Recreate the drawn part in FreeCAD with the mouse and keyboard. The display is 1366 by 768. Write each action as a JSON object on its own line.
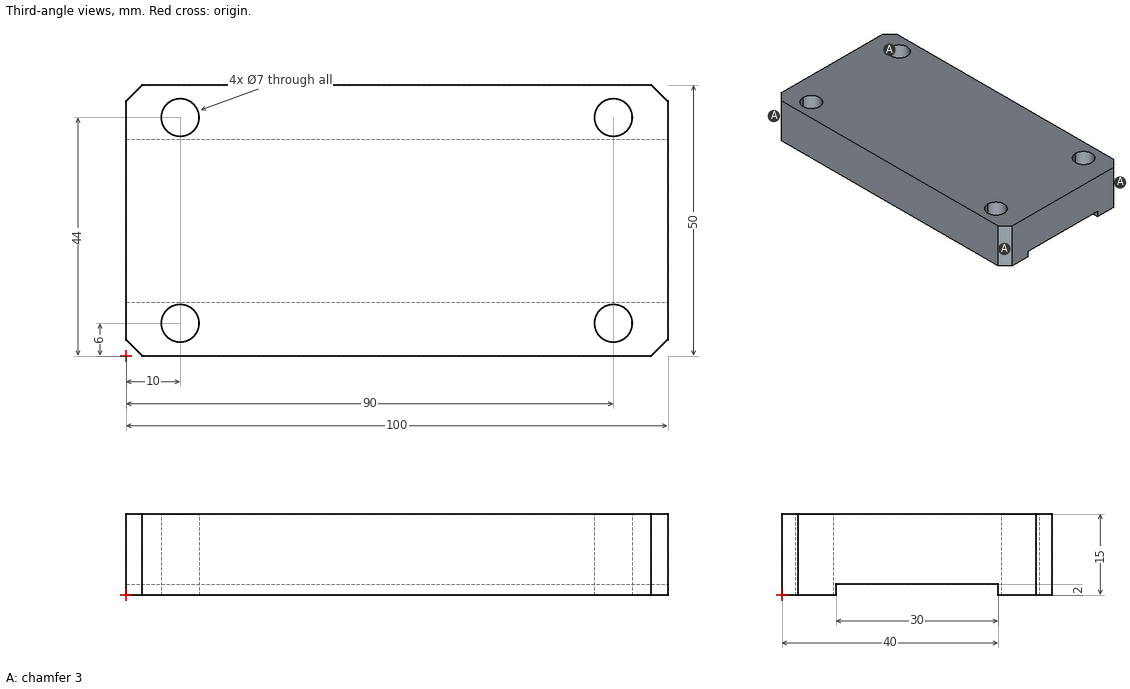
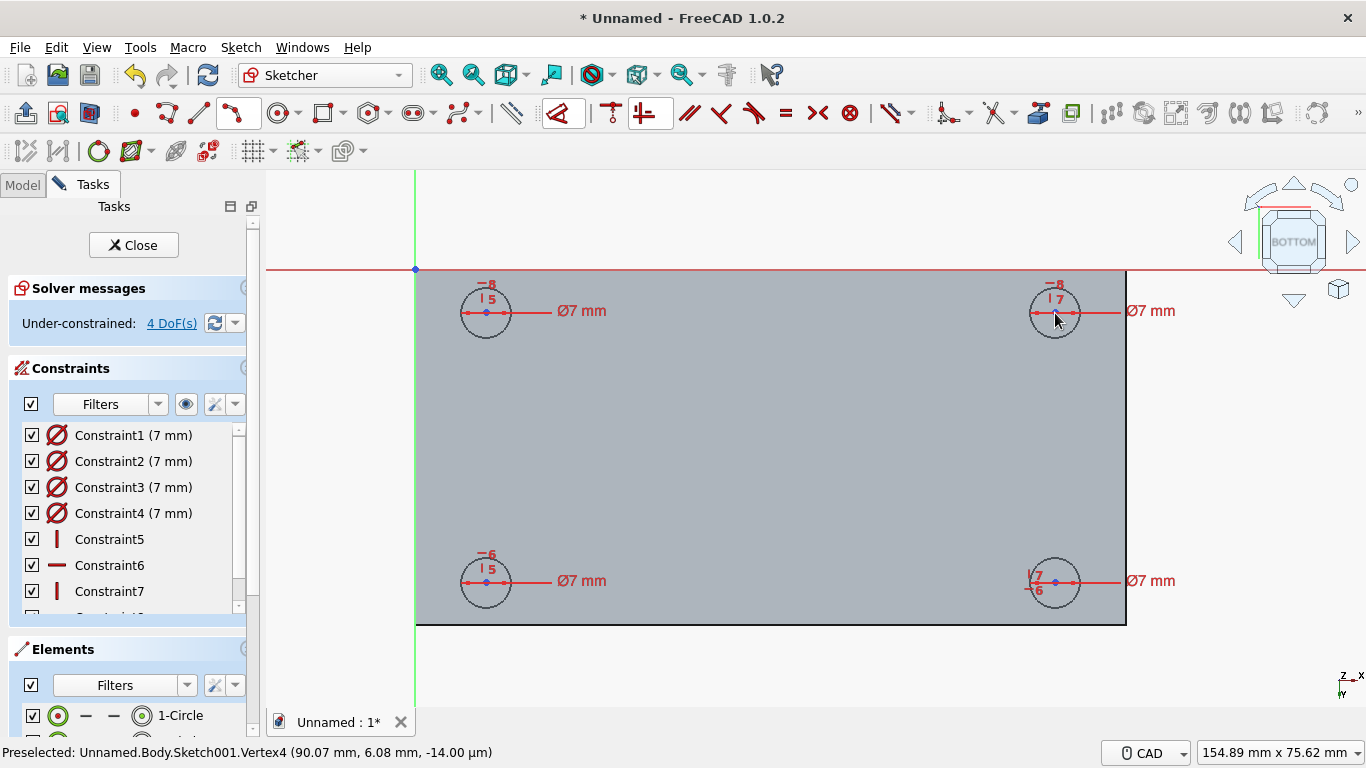
{"action": "left_click", "coordinate": [558, 114]}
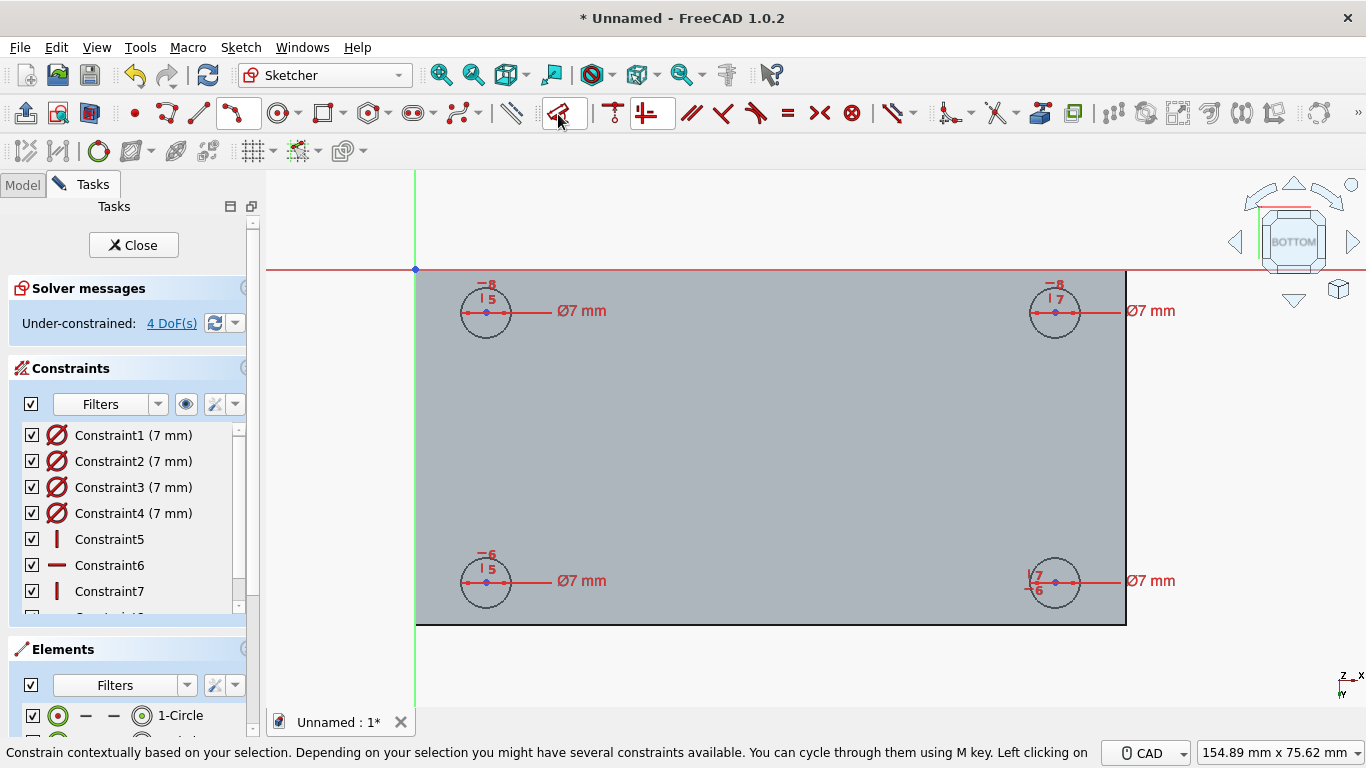
{"action": "left_click", "coordinate": [486, 313]}
{"action": "left_click", "coordinate": [381, 291]}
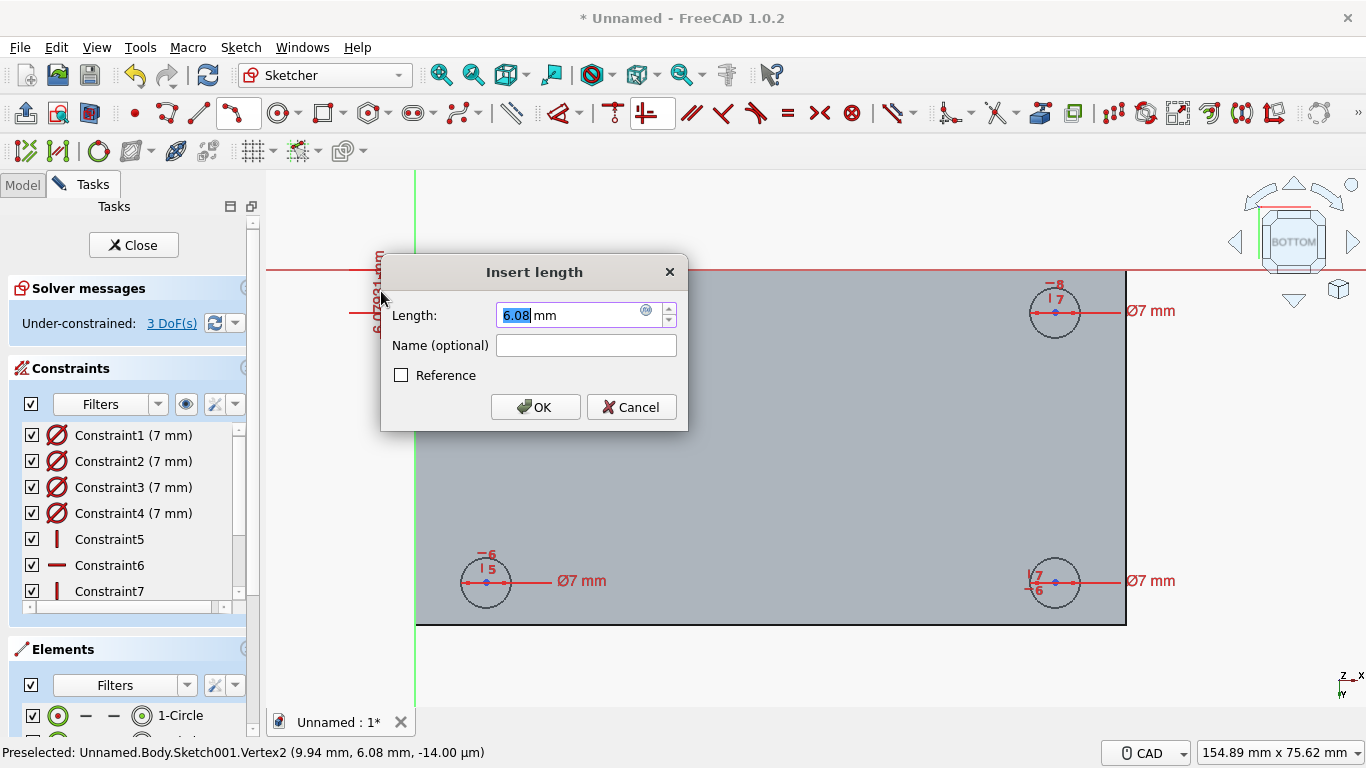
{"action": "type", "text": "6"}
{"action": "key", "text": "Return"}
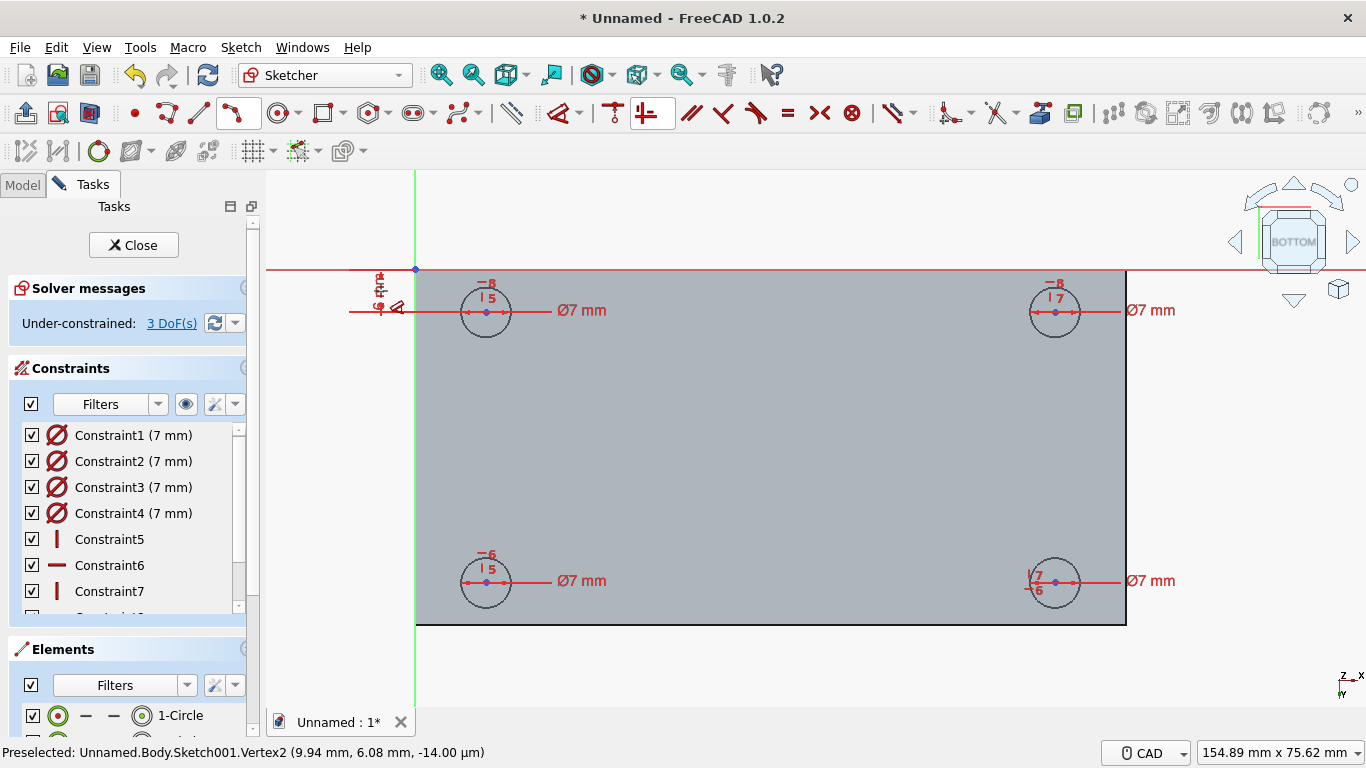
{"action": "left_click", "coordinate": [486, 583]}
{"action": "left_click", "coordinate": [451, 236]}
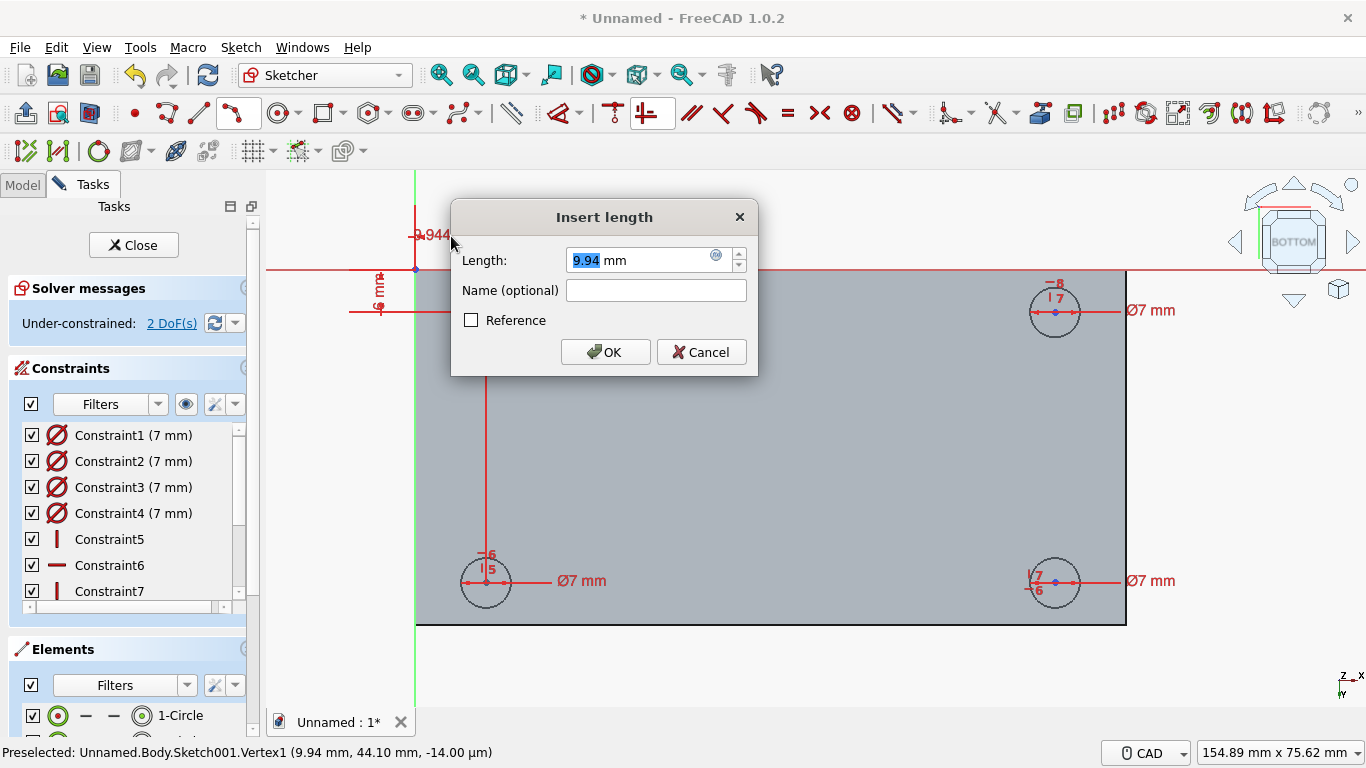
{"action": "type", "text": "10"}
{"action": "key", "text": "Return"}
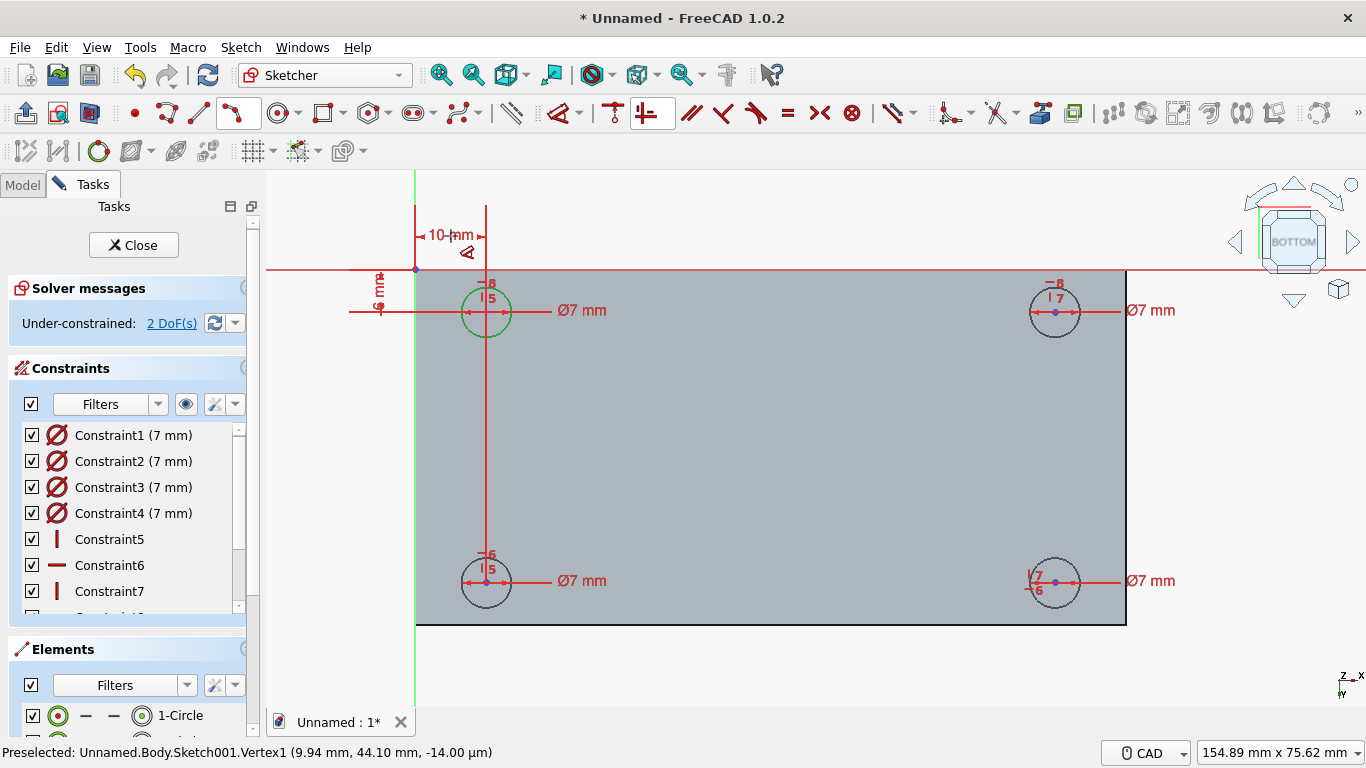
{"action": "left_click", "coordinate": [486, 583]}
{"action": "left_click", "coordinate": [381, 426]}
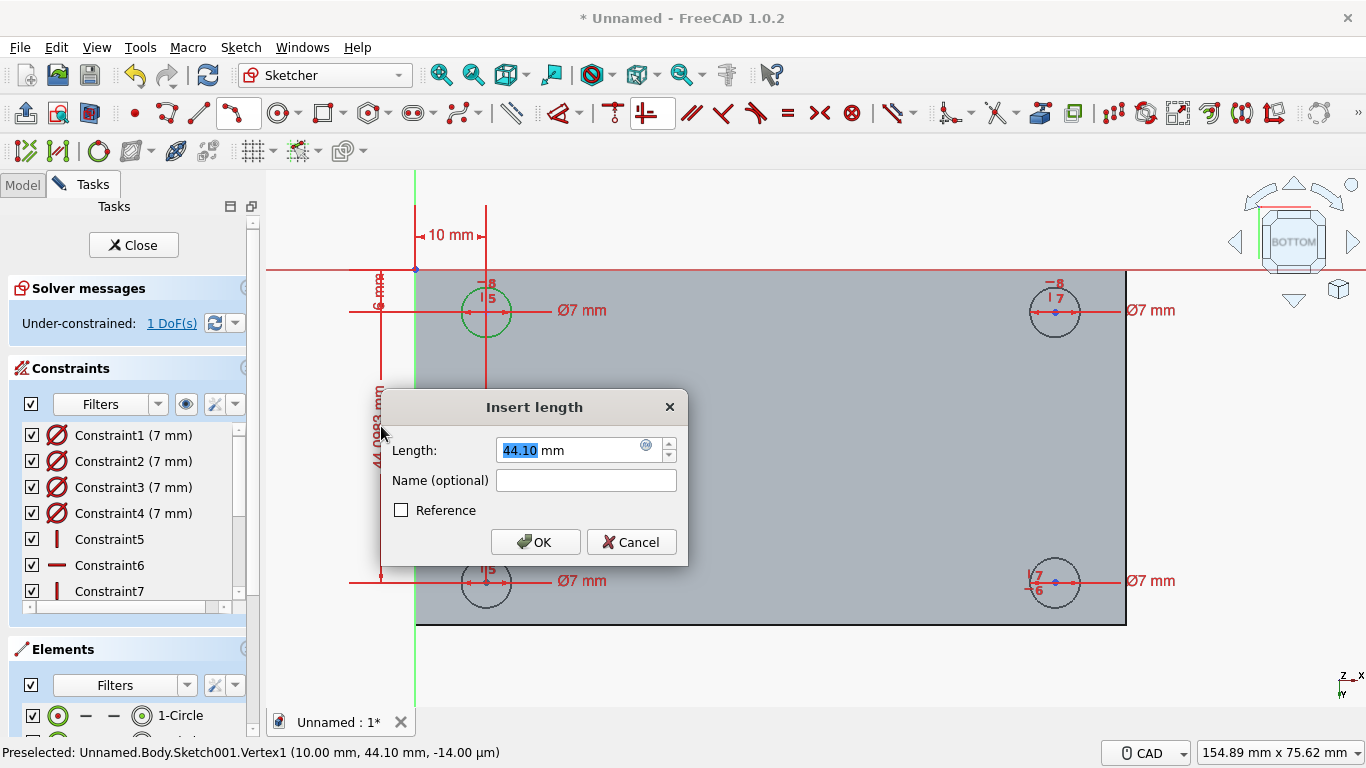
{"action": "type", "text": "44"}
{"action": "key", "text": "Return"}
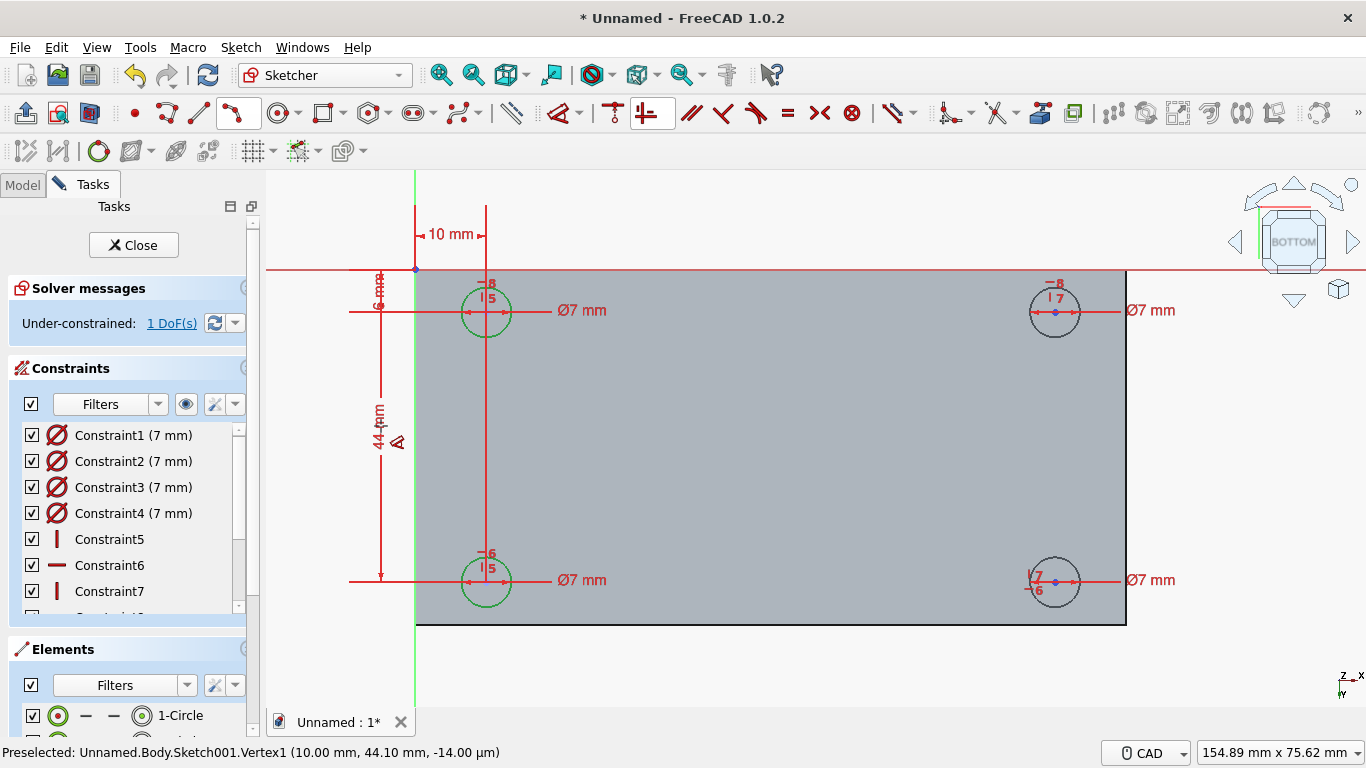
{"action": "left_click", "coordinate": [1055, 582]}
{"action": "left_click", "coordinate": [735, 236]}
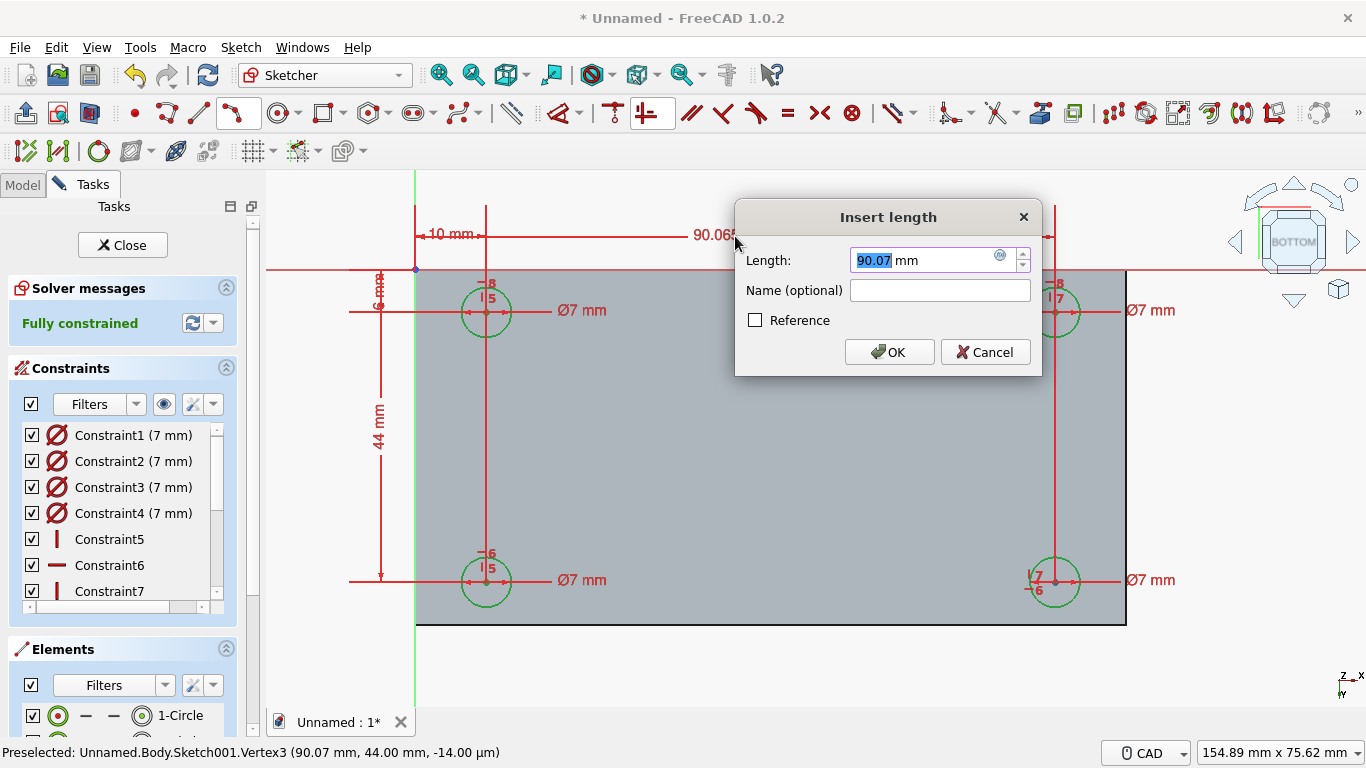
{"action": "type", "text": "90"}
{"action": "key", "text": "Return"}
{"action": "key", "text": "Escape"}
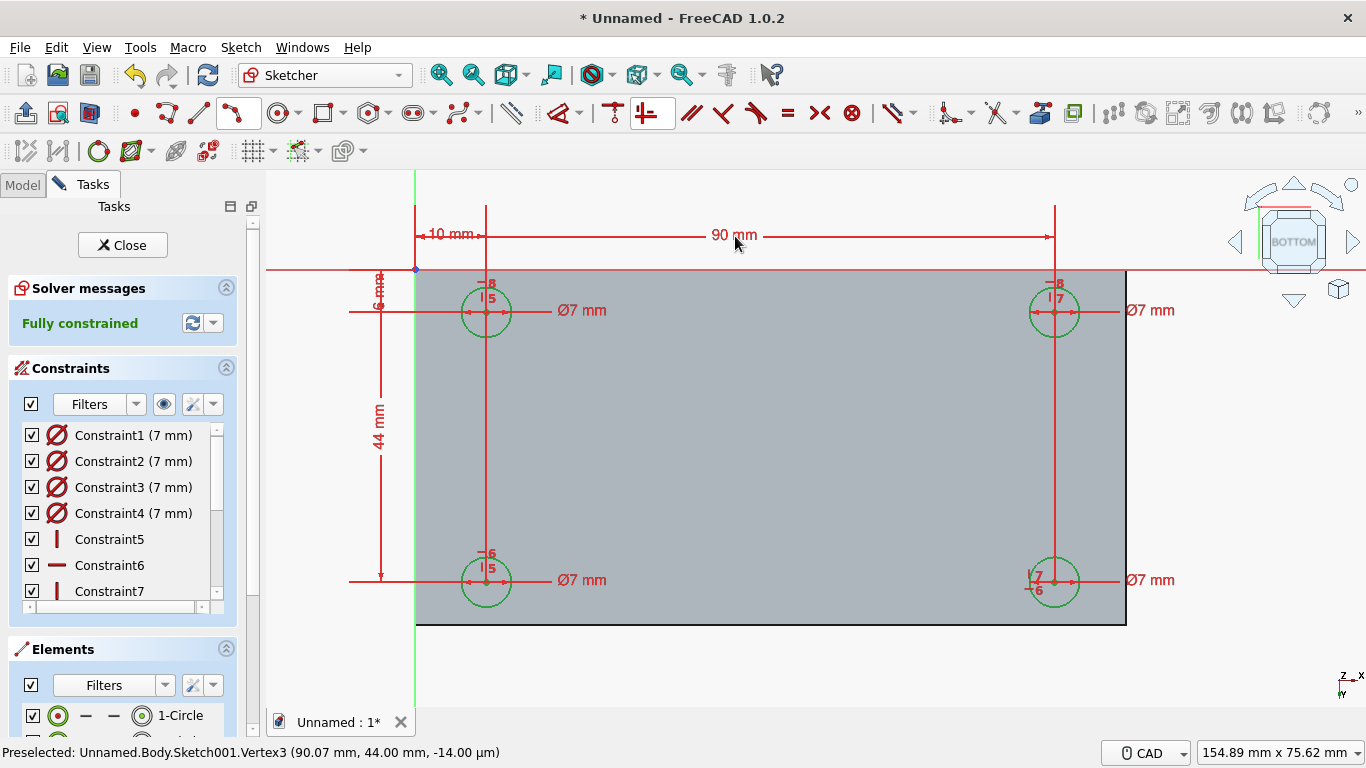
{"action": "left_click", "coordinate": [123, 245]}